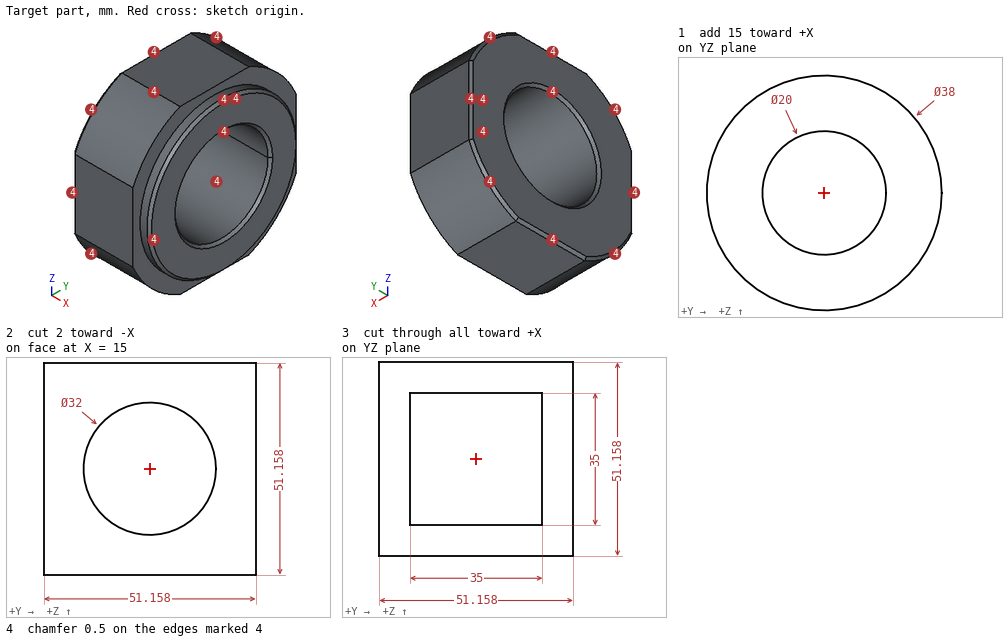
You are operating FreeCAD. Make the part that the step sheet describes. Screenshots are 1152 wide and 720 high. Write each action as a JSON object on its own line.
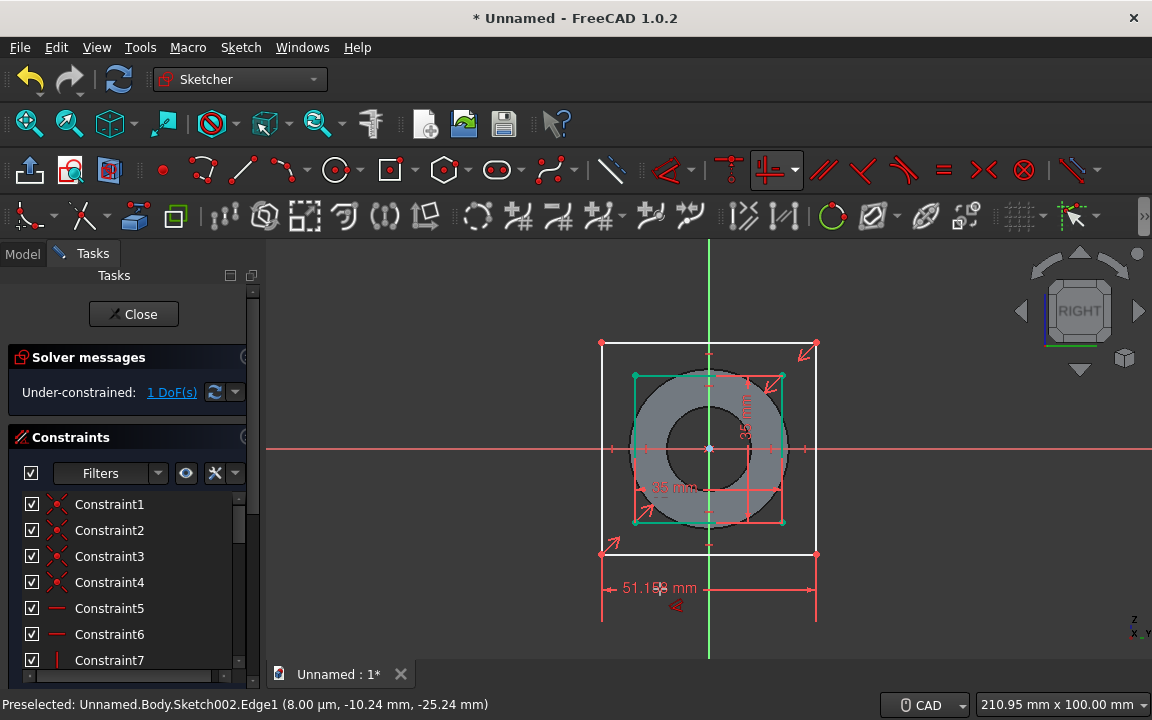
{"action": "left_click", "coordinate": [816, 491]}
{"action": "left_click", "coordinate": [850, 400]}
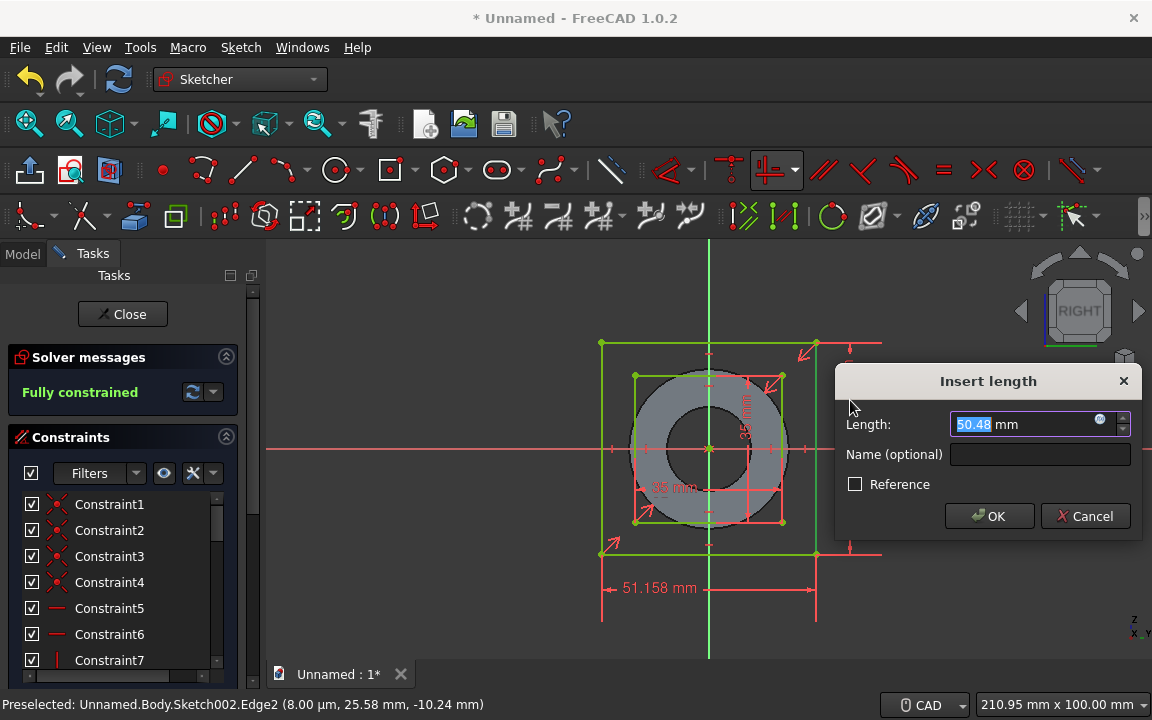
{"action": "type", "text": "51.158"}
{"action": "key", "text": "Return"}
{"action": "key", "text": "Escape"}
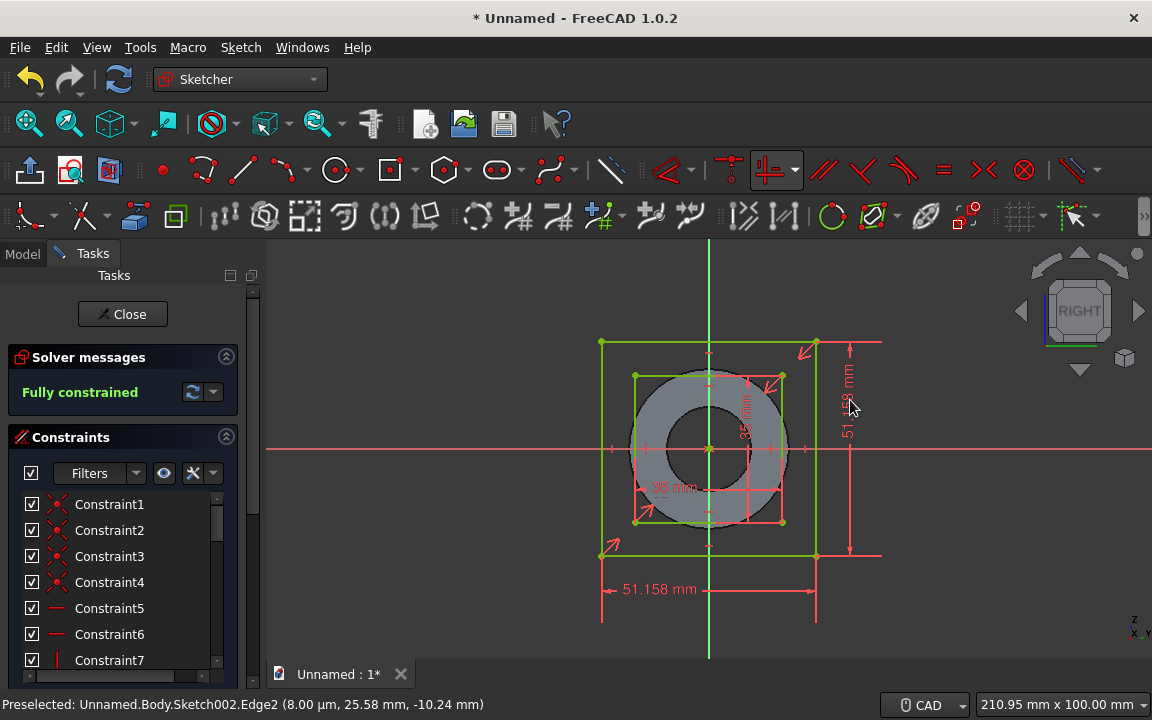
{"action": "left_click", "coordinate": [123, 314]}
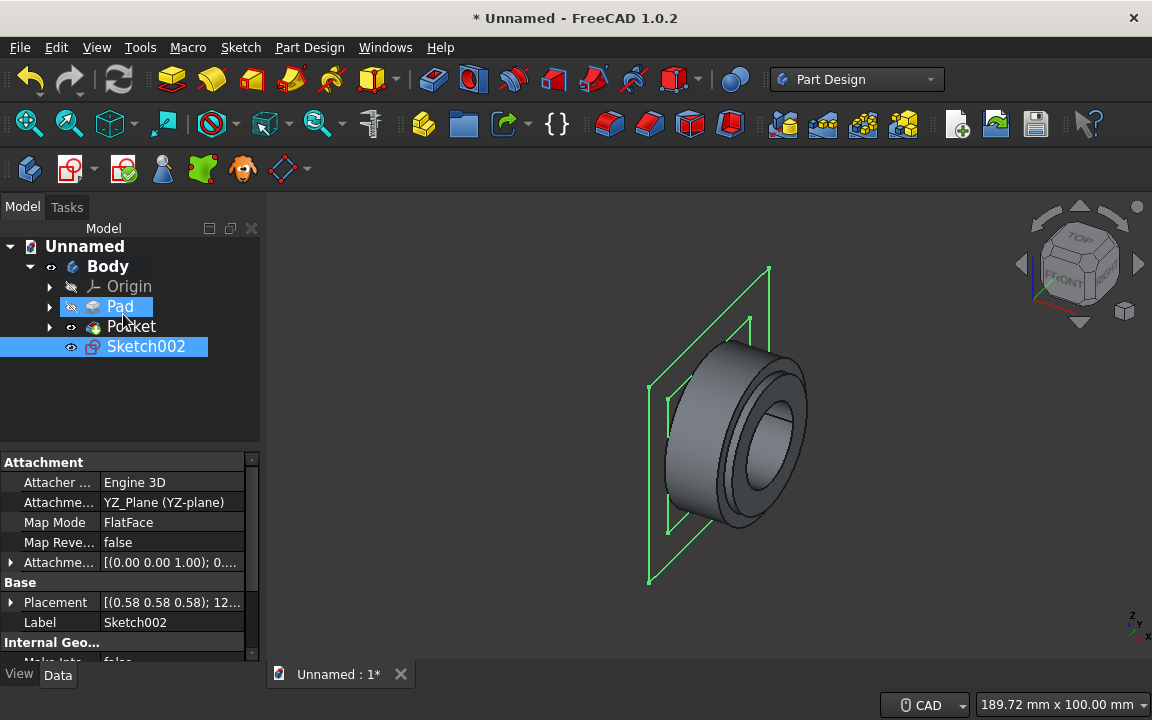
{"action": "left_click", "coordinate": [434, 80]}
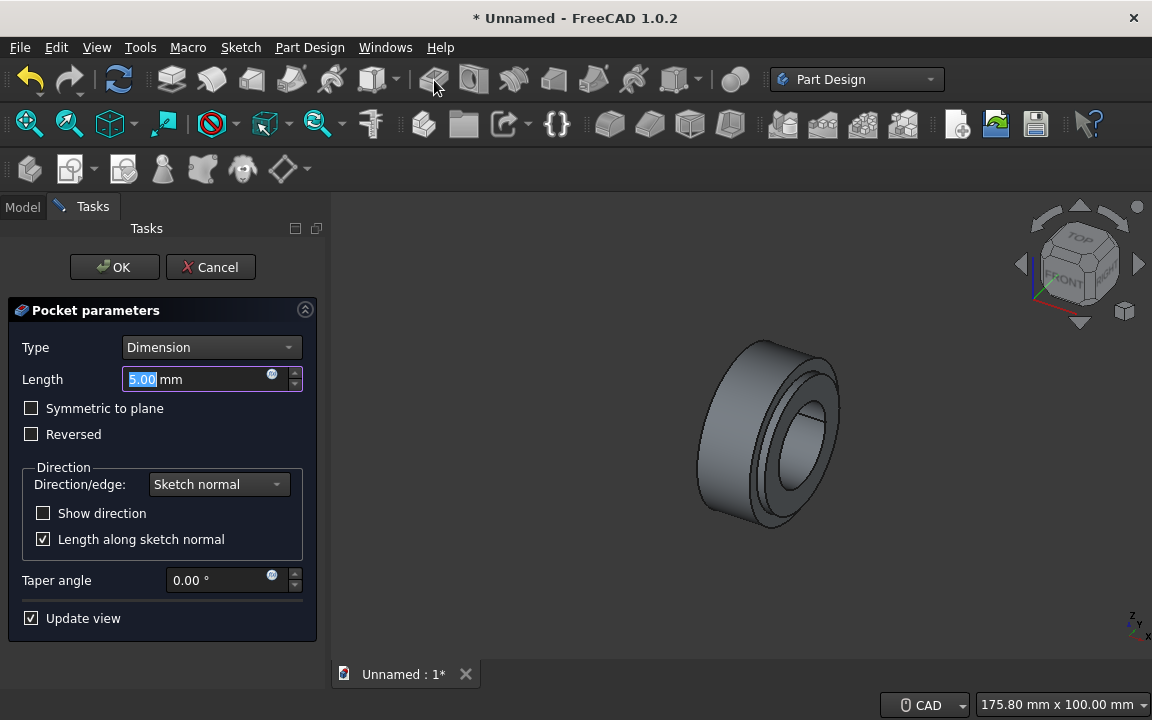
{"action": "left_click", "coordinate": [212, 348]}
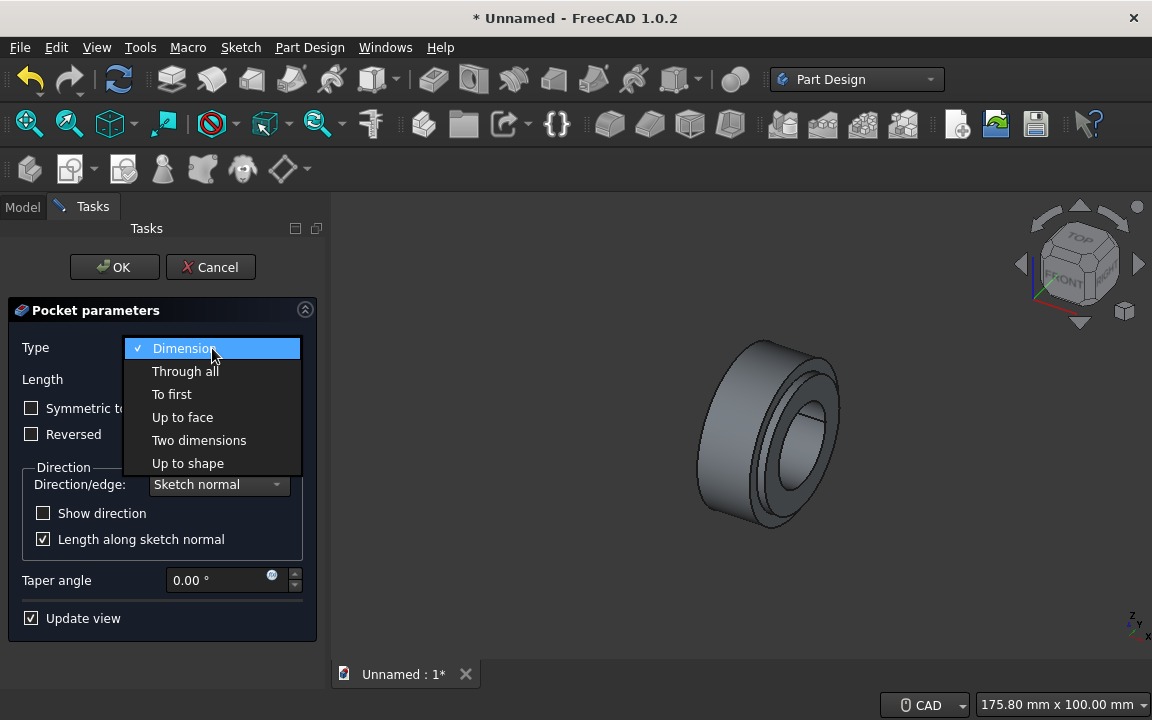
{"action": "left_click", "coordinate": [212, 372]}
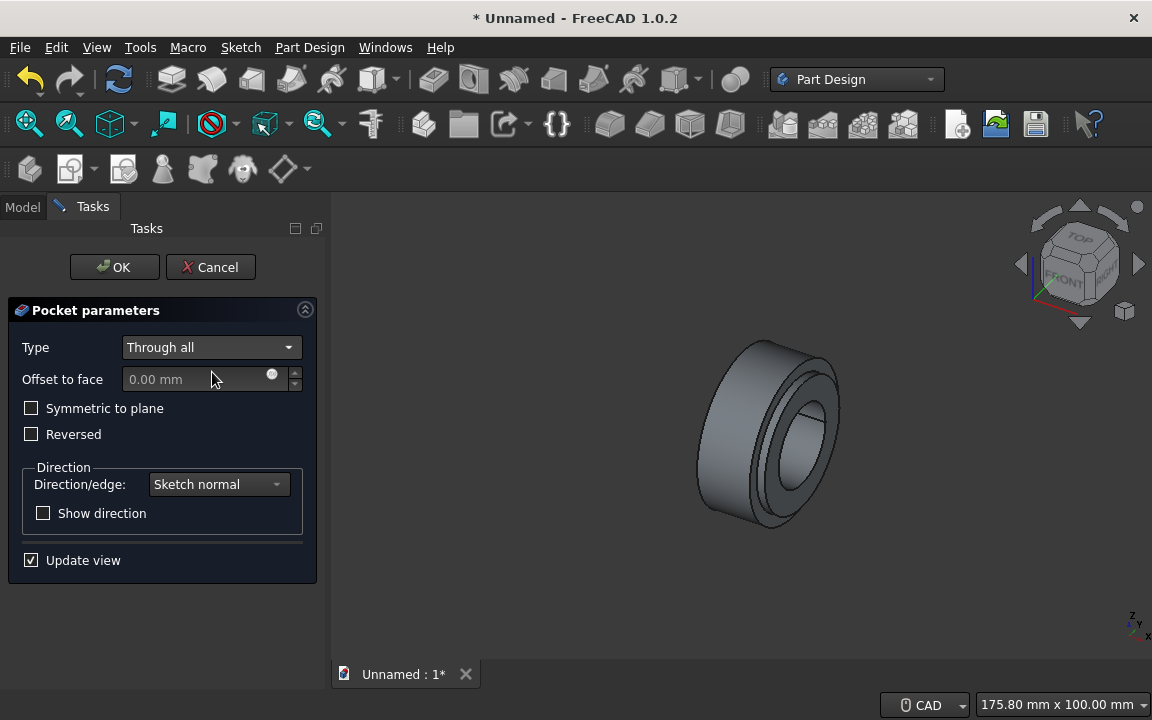
{"action": "left_click", "coordinate": [30, 434]}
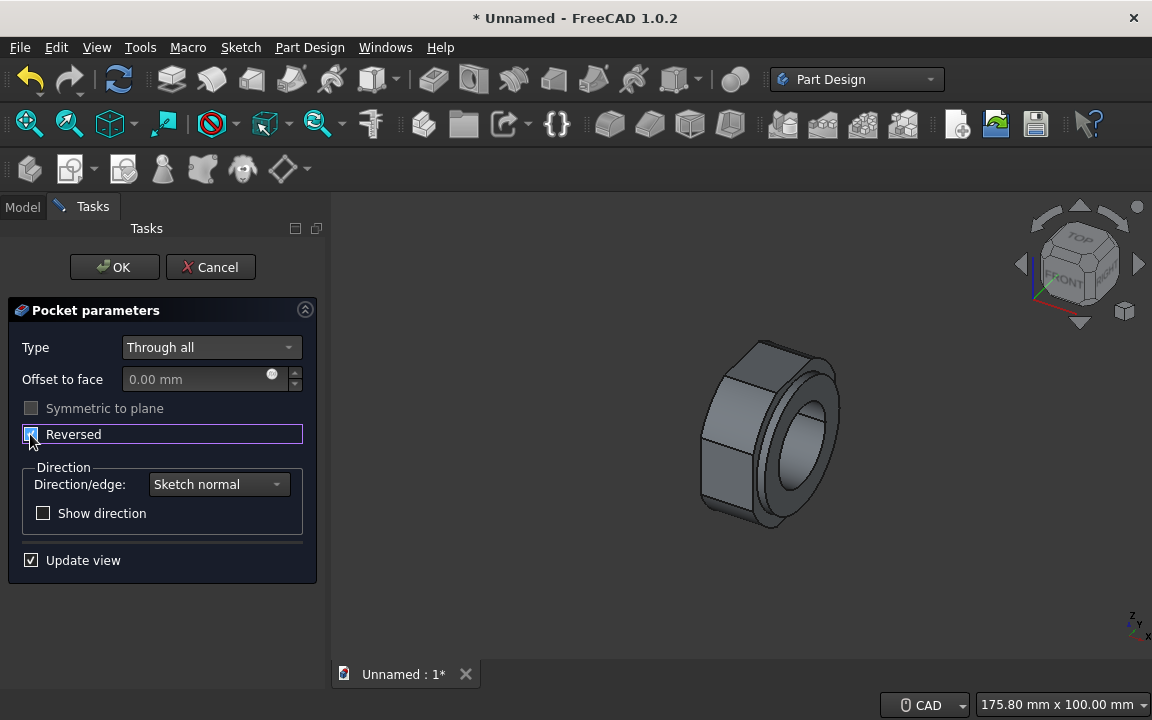
{"action": "left_click", "coordinate": [115, 267]}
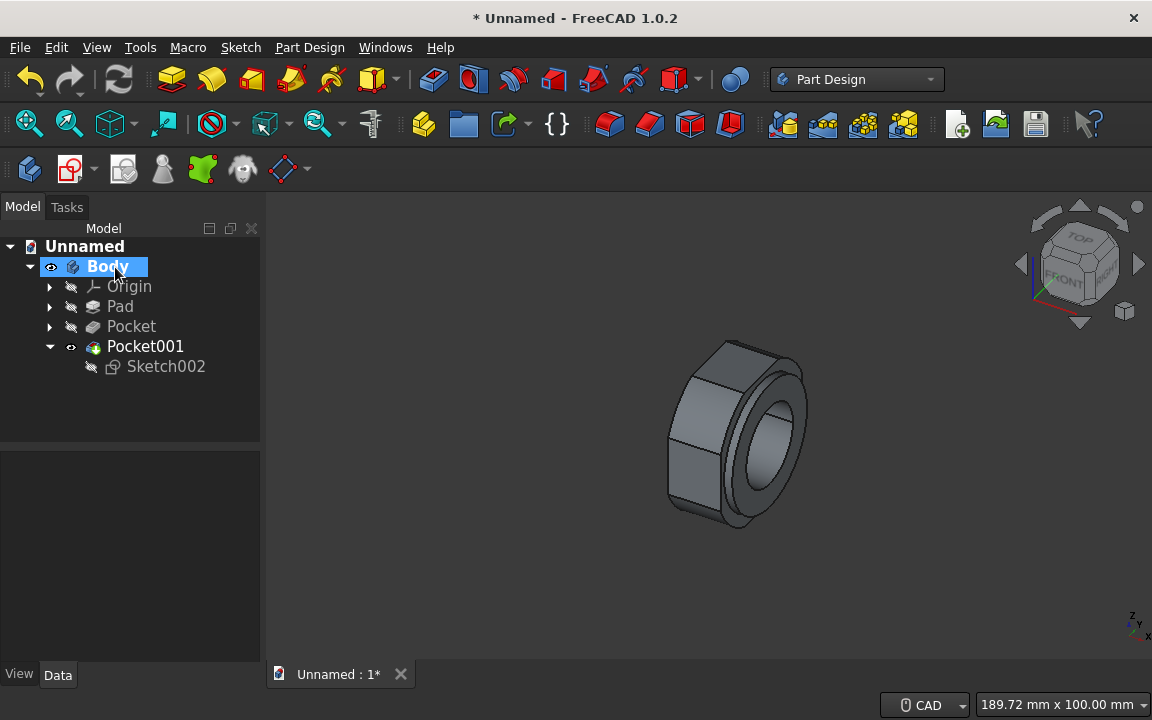
{"action": "left_click", "coordinate": [732, 482]}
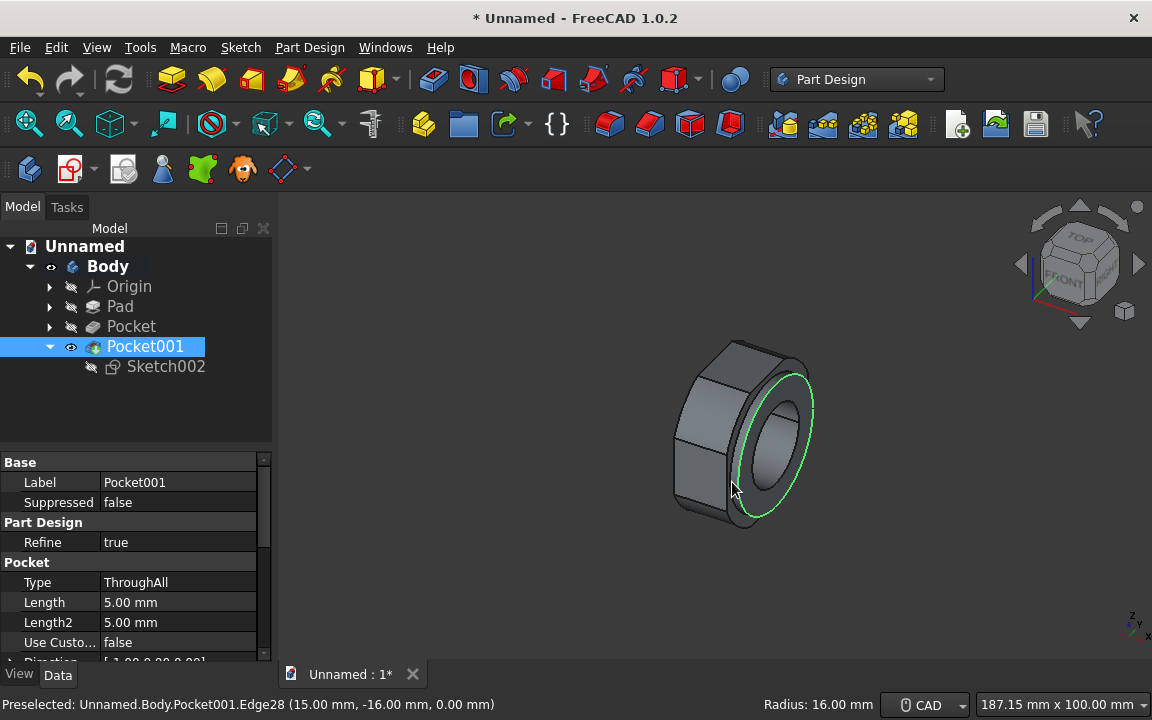
{"action": "left_click", "coordinate": [768, 488], "text": "ctrl"}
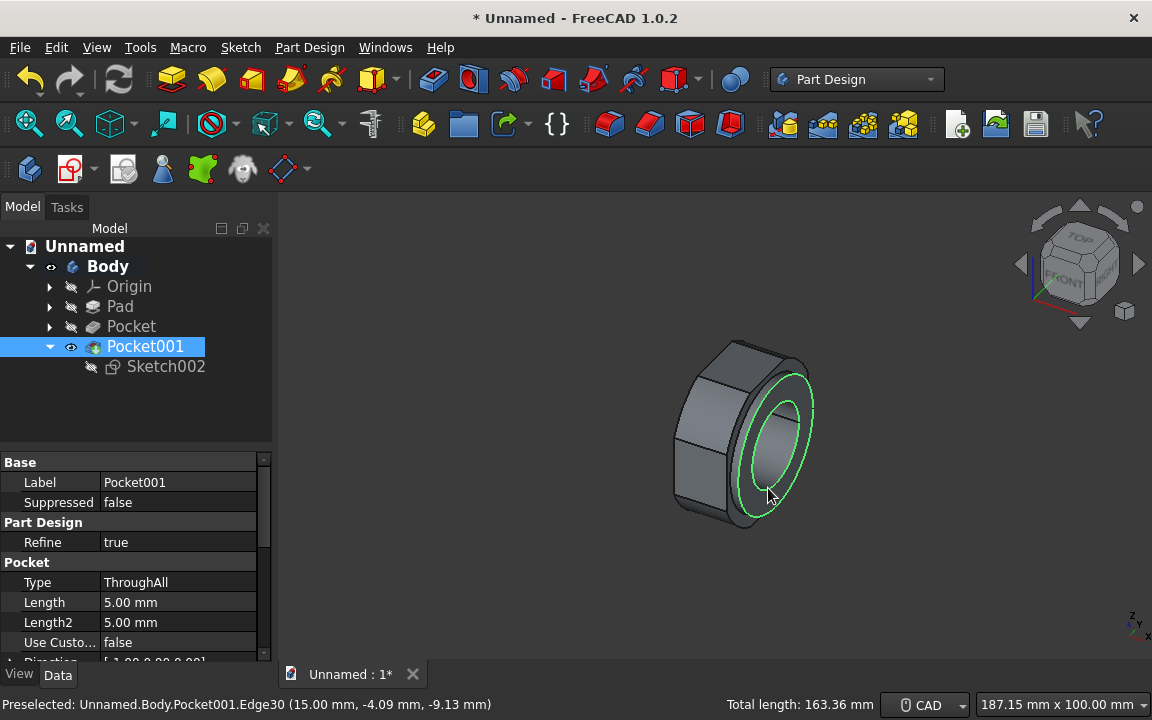
{"action": "key", "text": "0"}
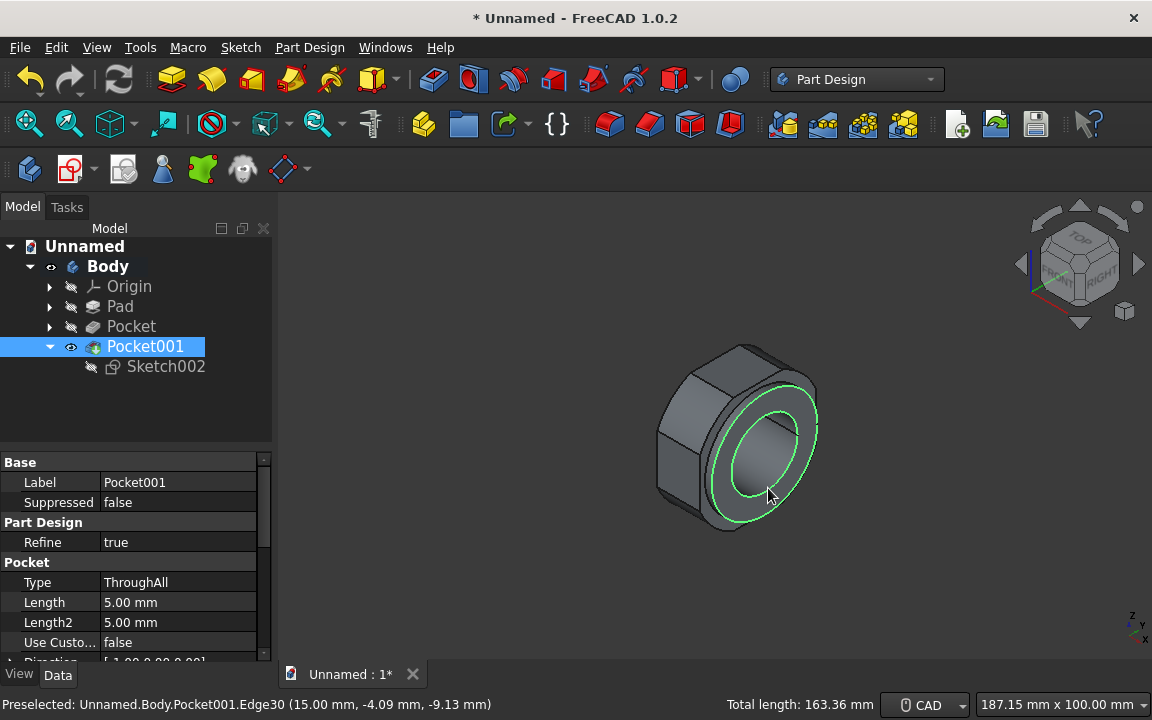
{"action": "key", "text": "2"}